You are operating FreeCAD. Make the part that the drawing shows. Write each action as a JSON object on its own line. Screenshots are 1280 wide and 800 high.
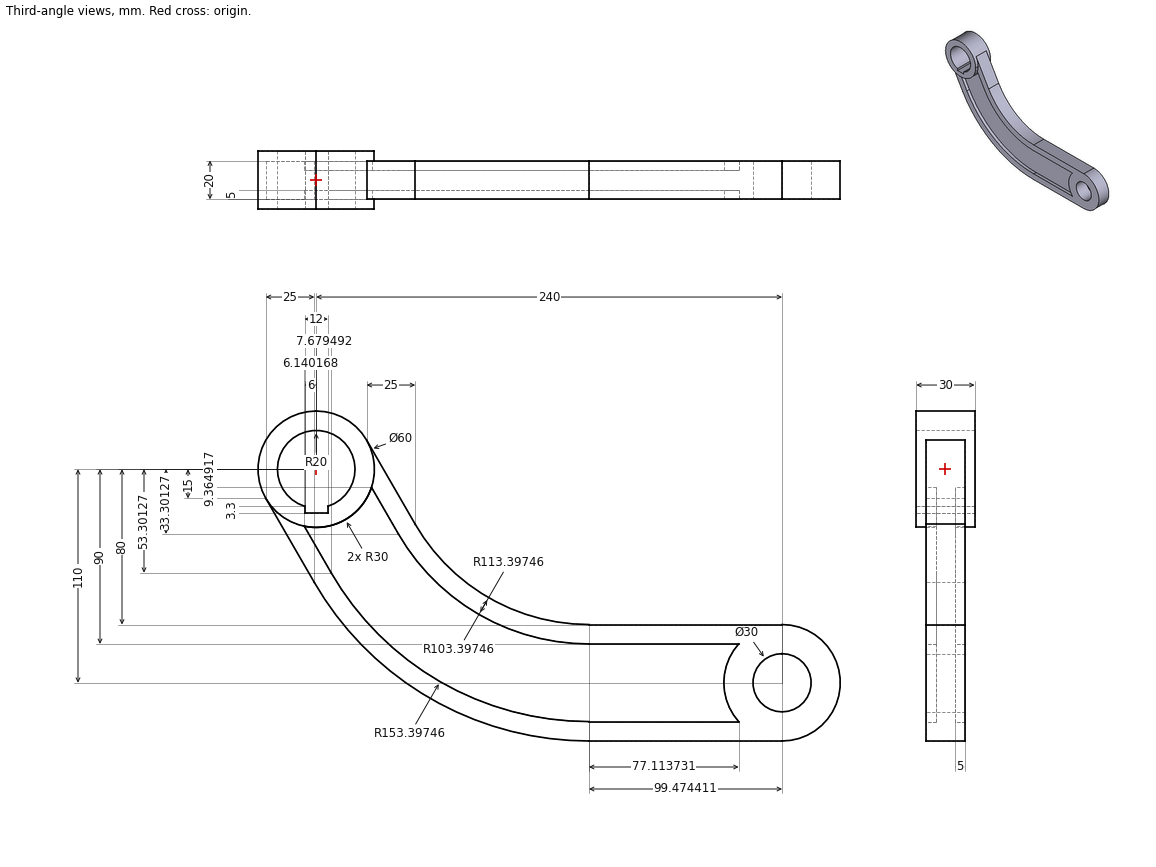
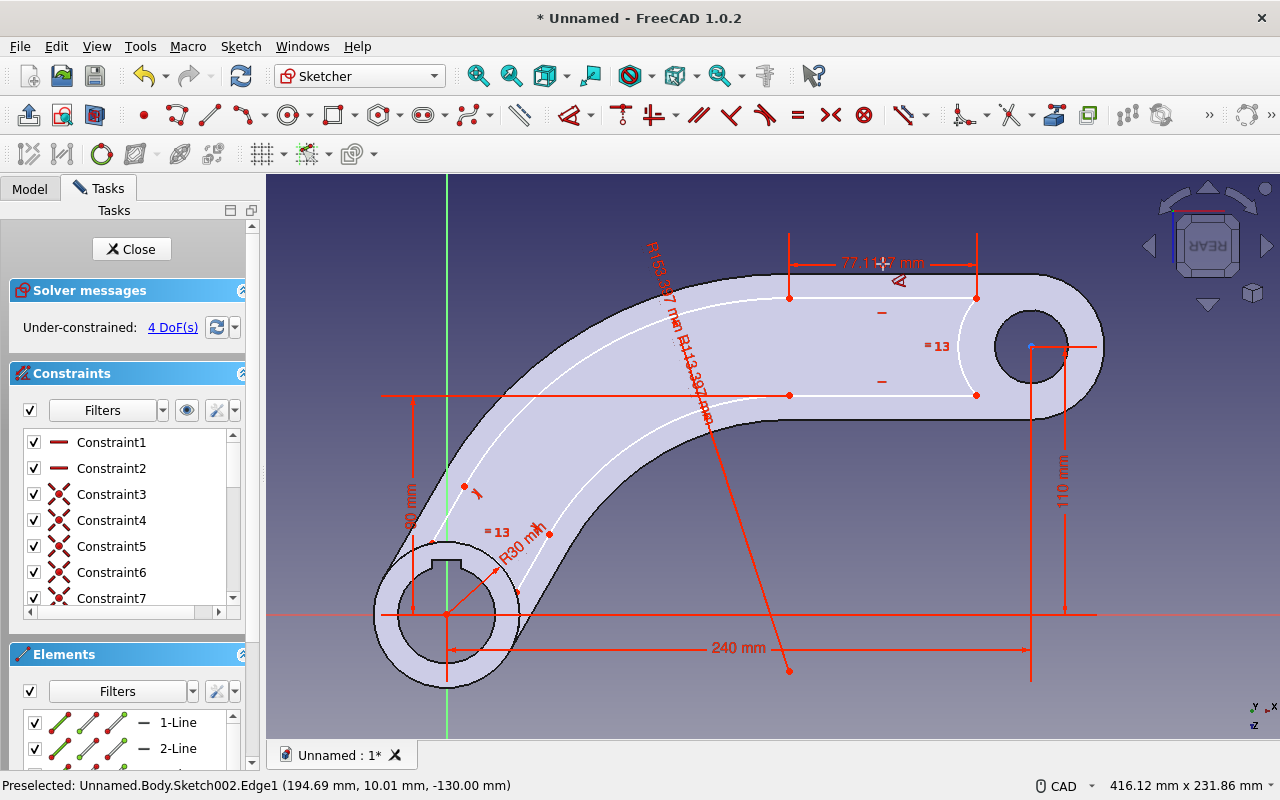
{"action": "left_click", "coordinate": [845, 396]}
{"action": "left_click", "coordinate": [883, 362]}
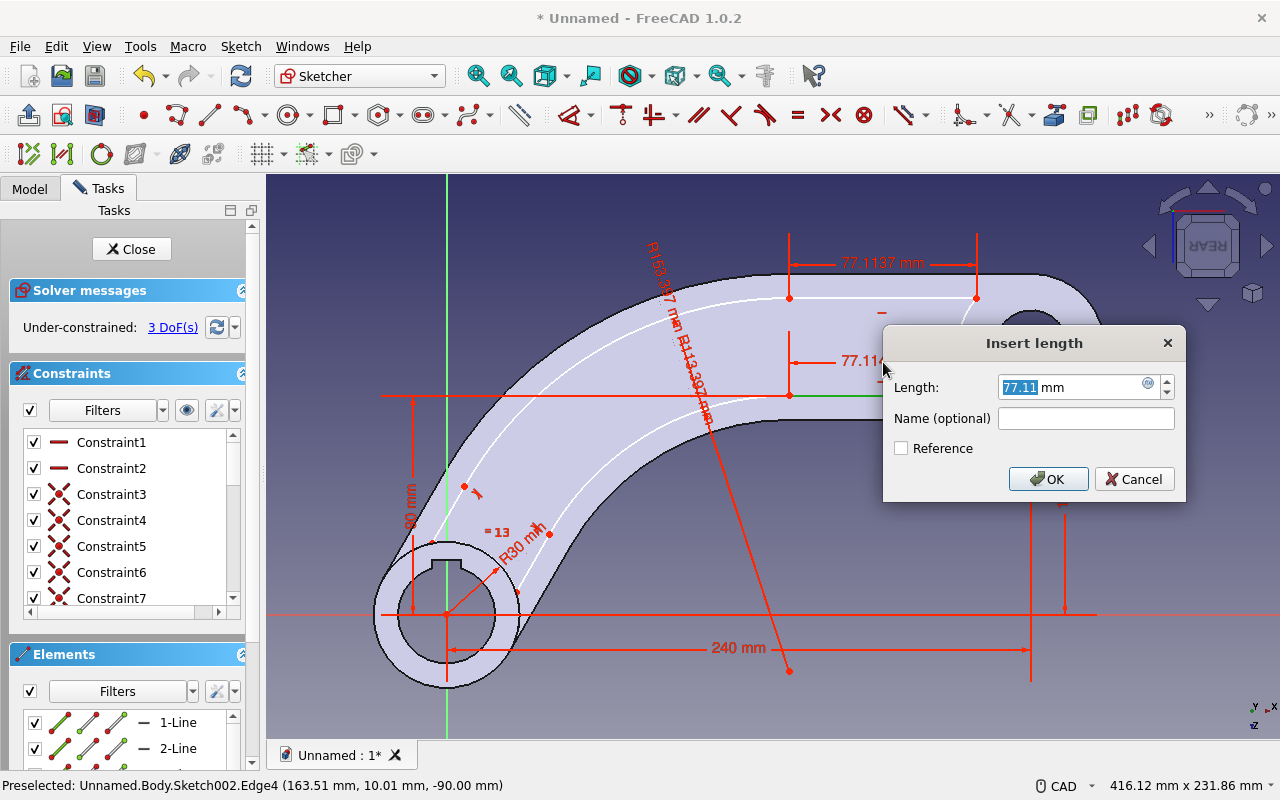
{"action": "type", "text": "77.113731"}
{"action": "key", "text": "Return"}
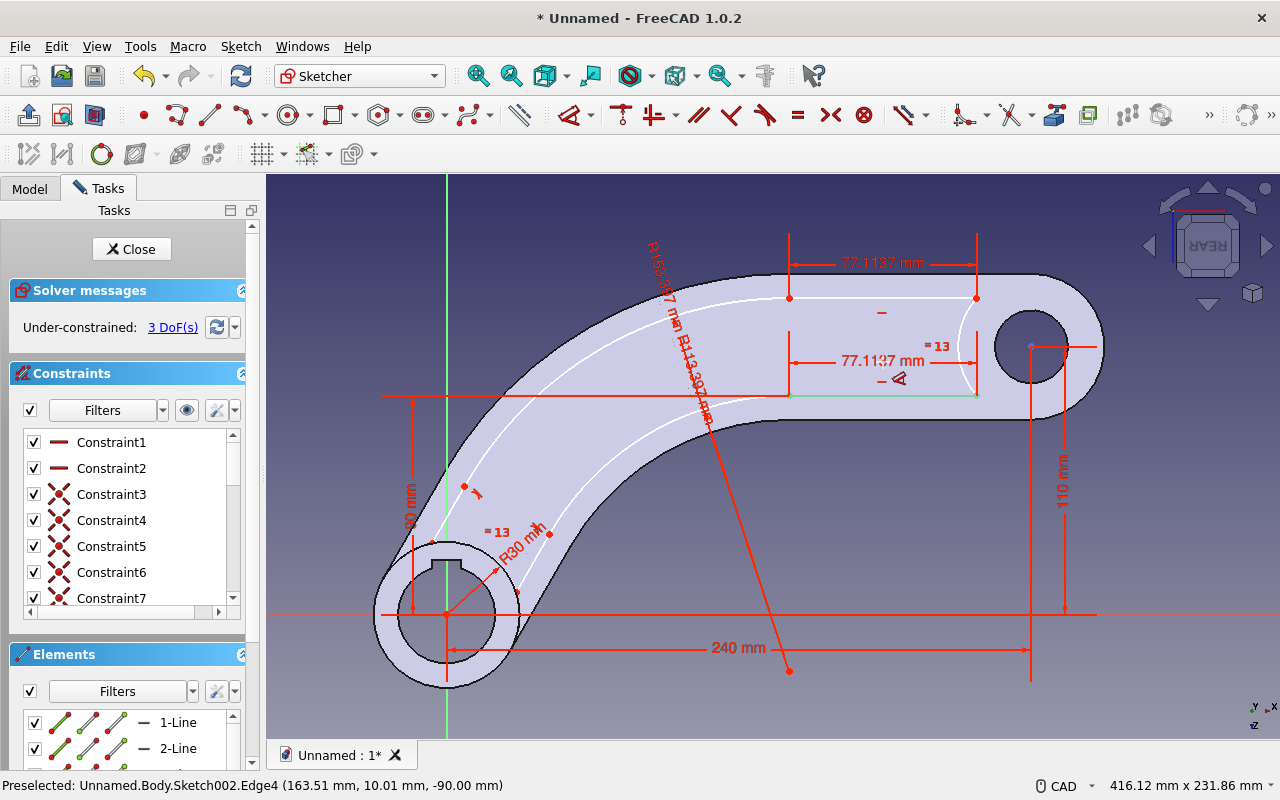
{"action": "scroll", "coordinate": [465, 486], "scroll_direction": "up", "scroll_amount": 4}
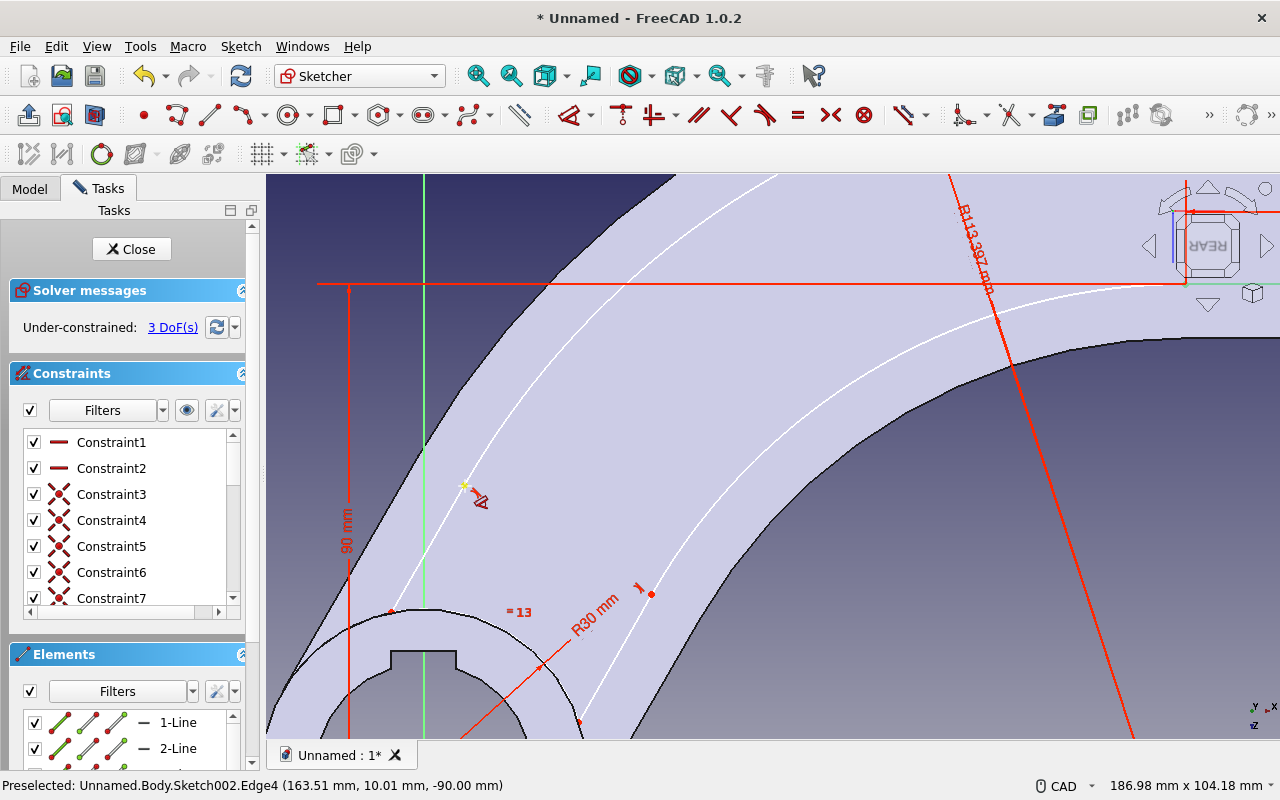
{"action": "left_click", "coordinate": [464, 485]}
{"action": "left_click", "coordinate": [444, 451]}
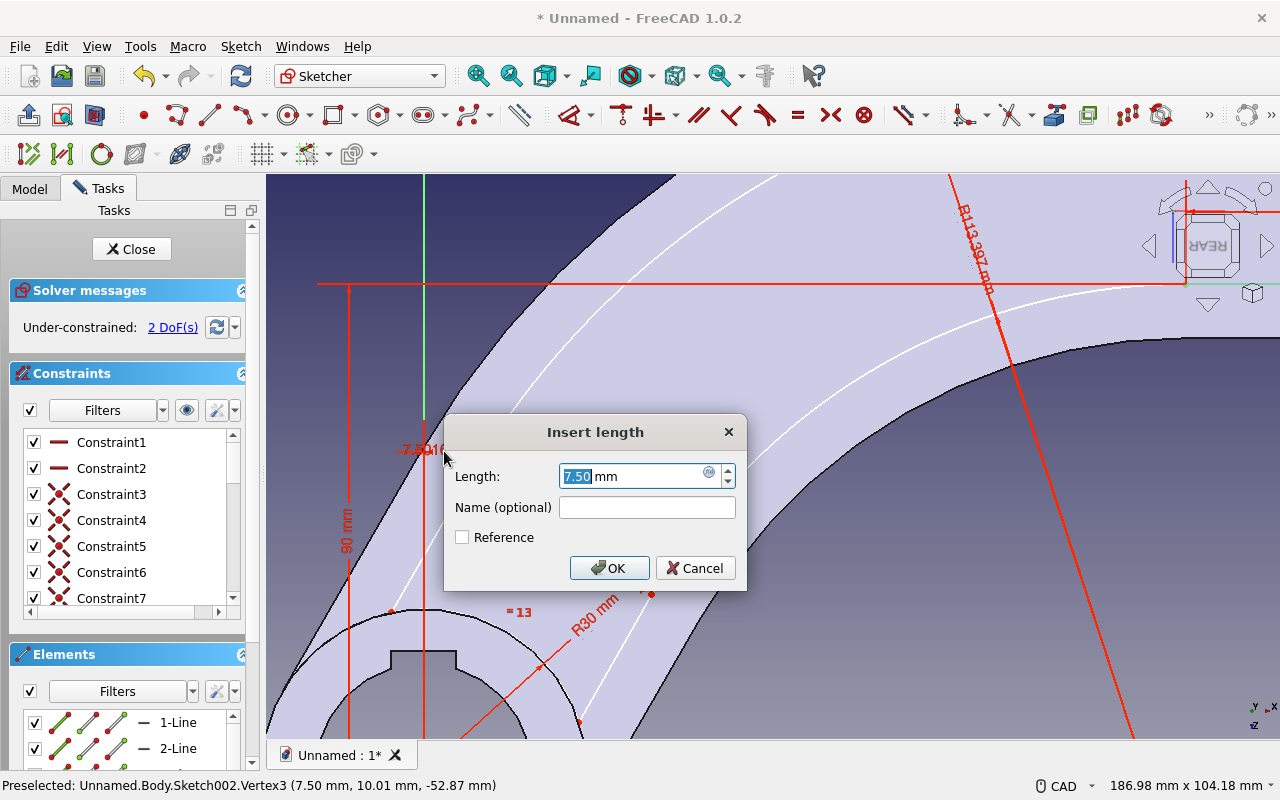
{"action": "type", "text": "7.679492"}
{"action": "key", "text": "Return"}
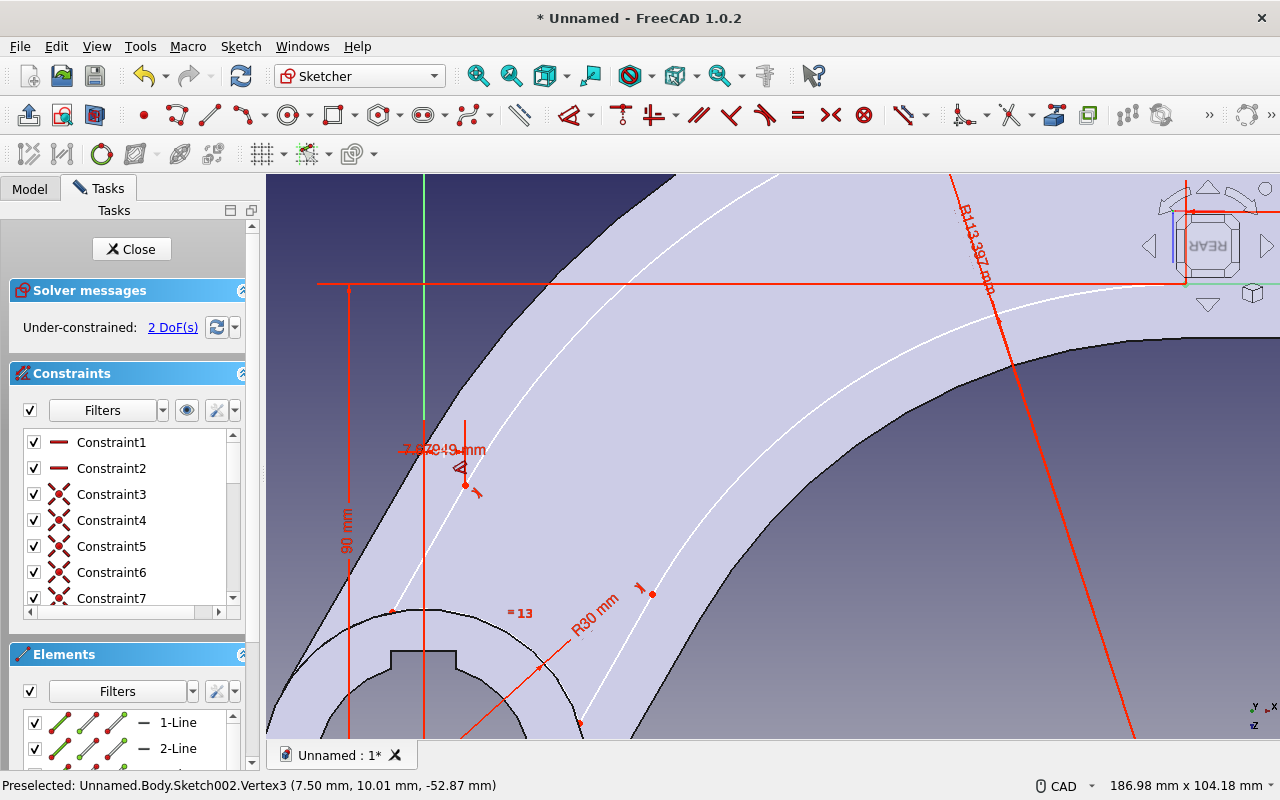
{"action": "left_click", "coordinate": [465, 485]}
{"action": "left_click", "coordinate": [390, 650]}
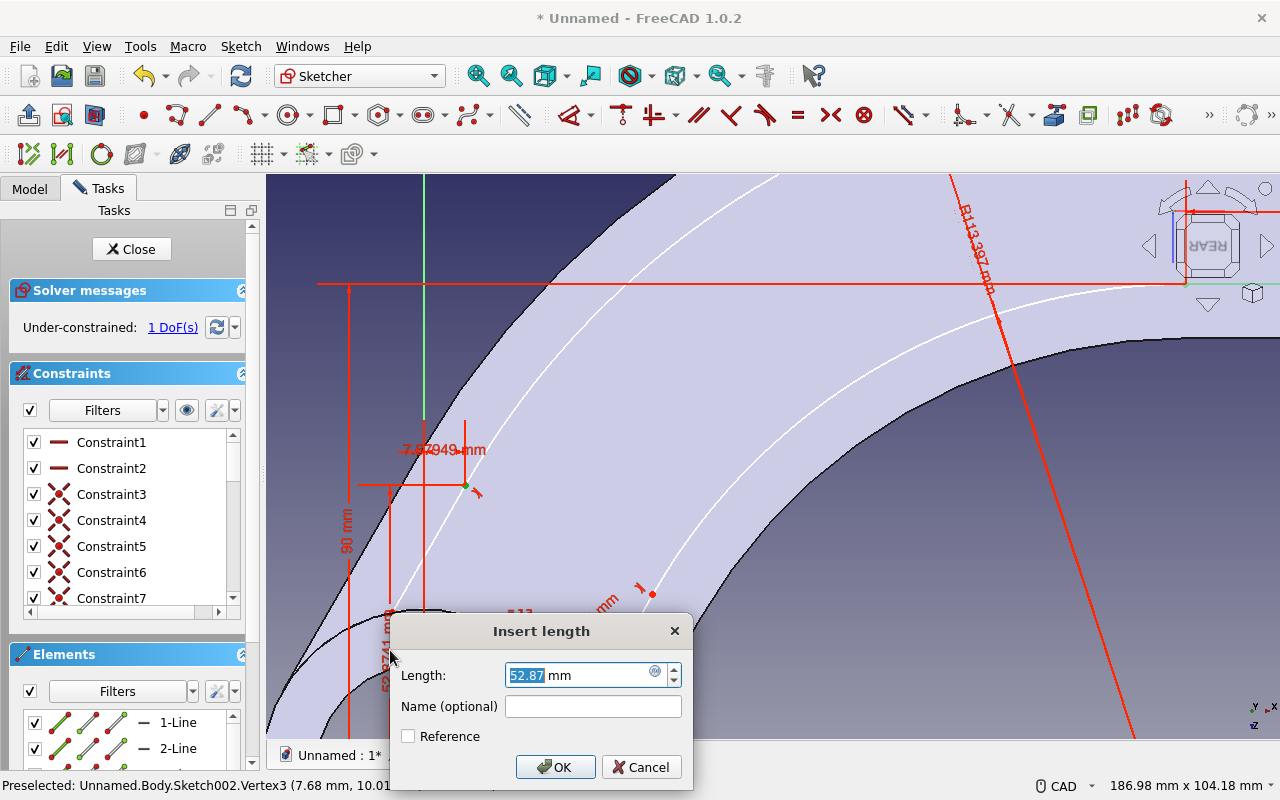
{"action": "type", "text": "53.30127"}
{"action": "key", "text": "Return"}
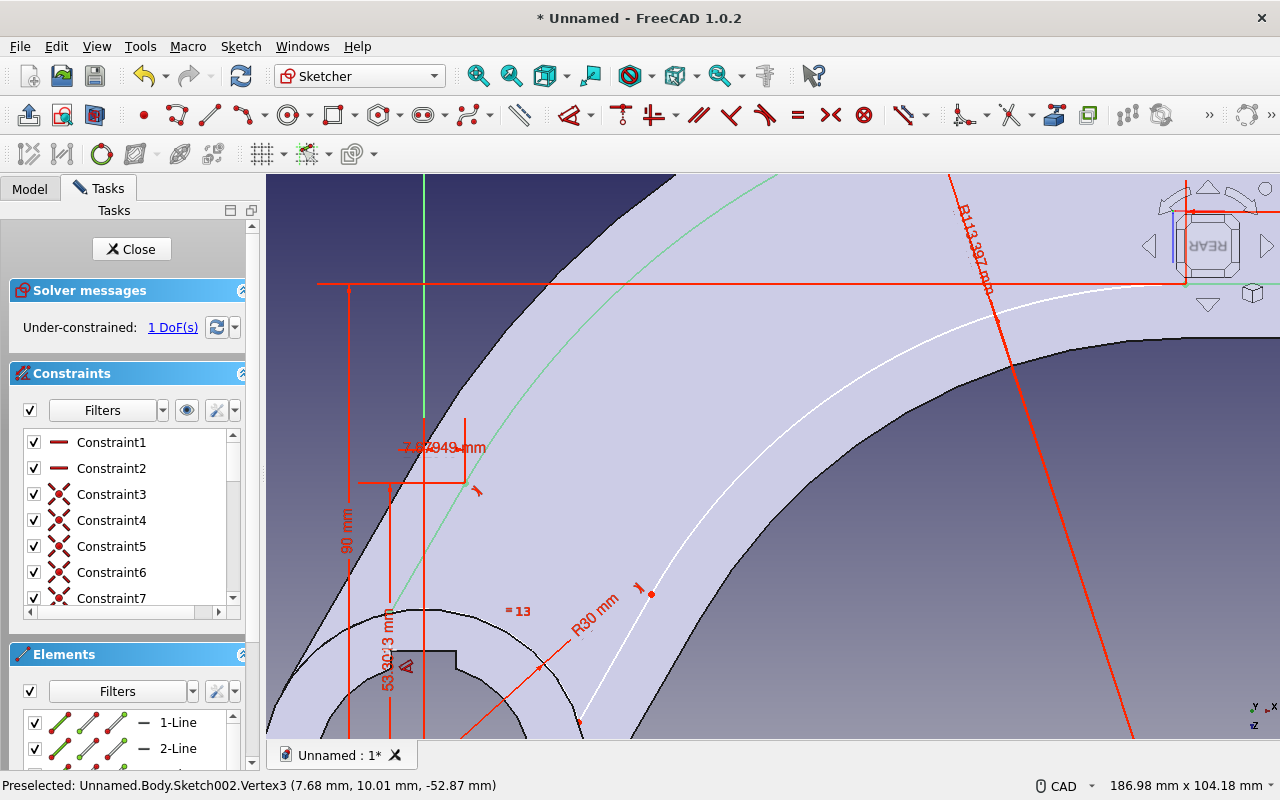
{"action": "scroll", "coordinate": [466, 487], "scroll_direction": "down", "scroll_amount": 4}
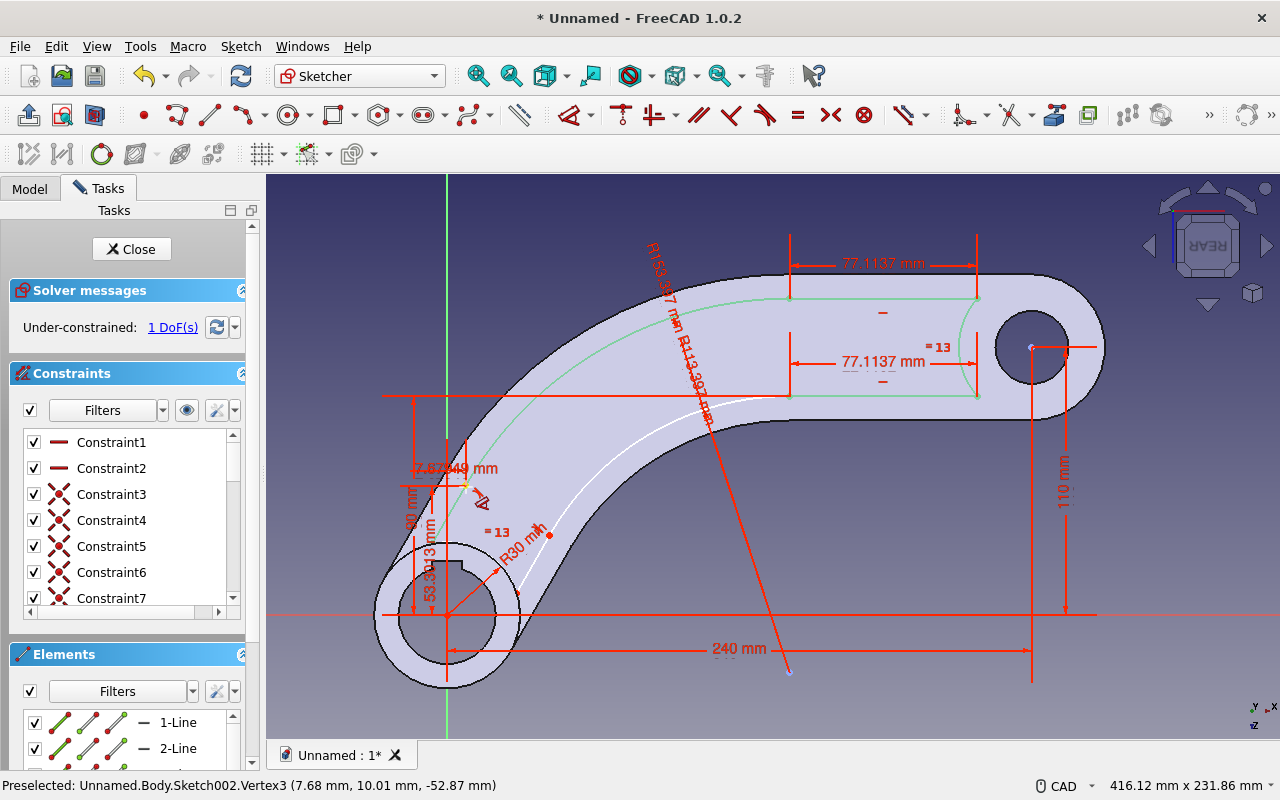
{"action": "scroll", "coordinate": [517, 593], "scroll_direction": "up", "scroll_amount": 3}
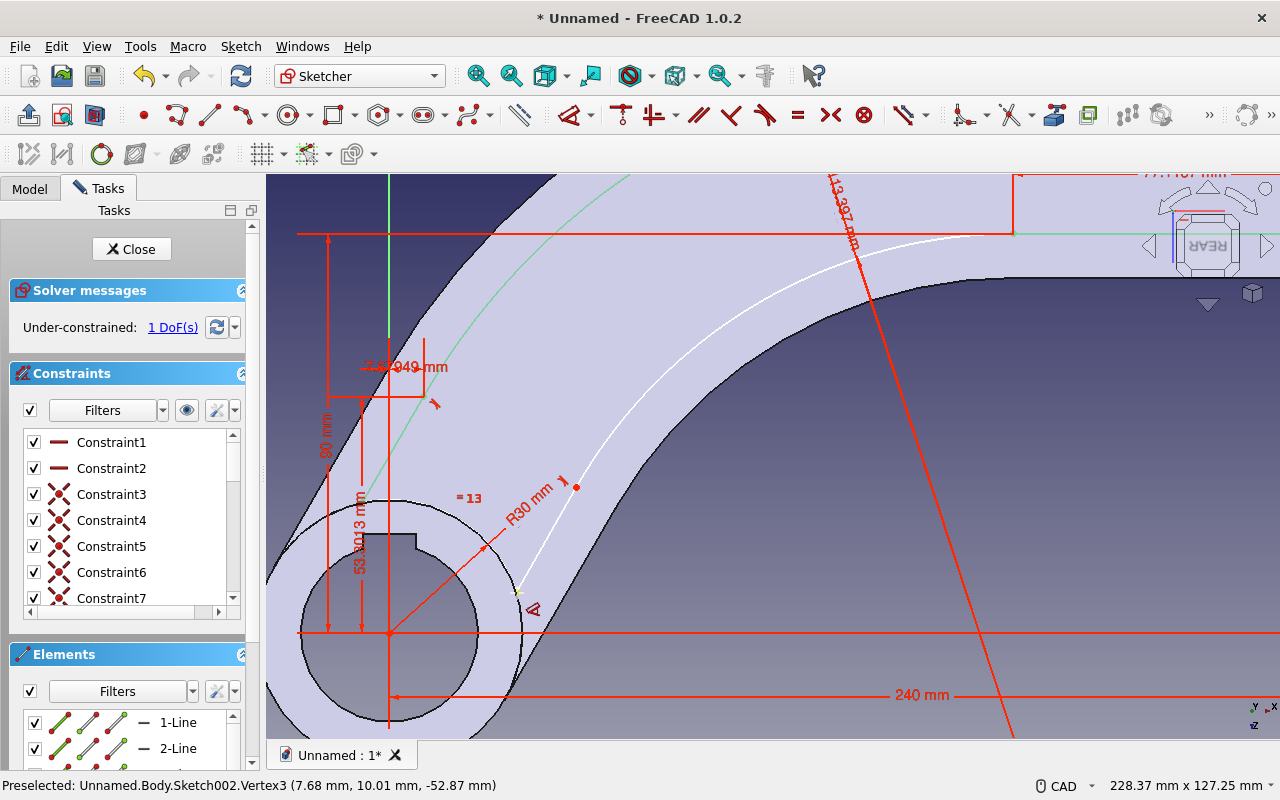
{"action": "left_click", "coordinate": [516, 592]}
{"action": "left_click", "coordinate": [355, 613]}